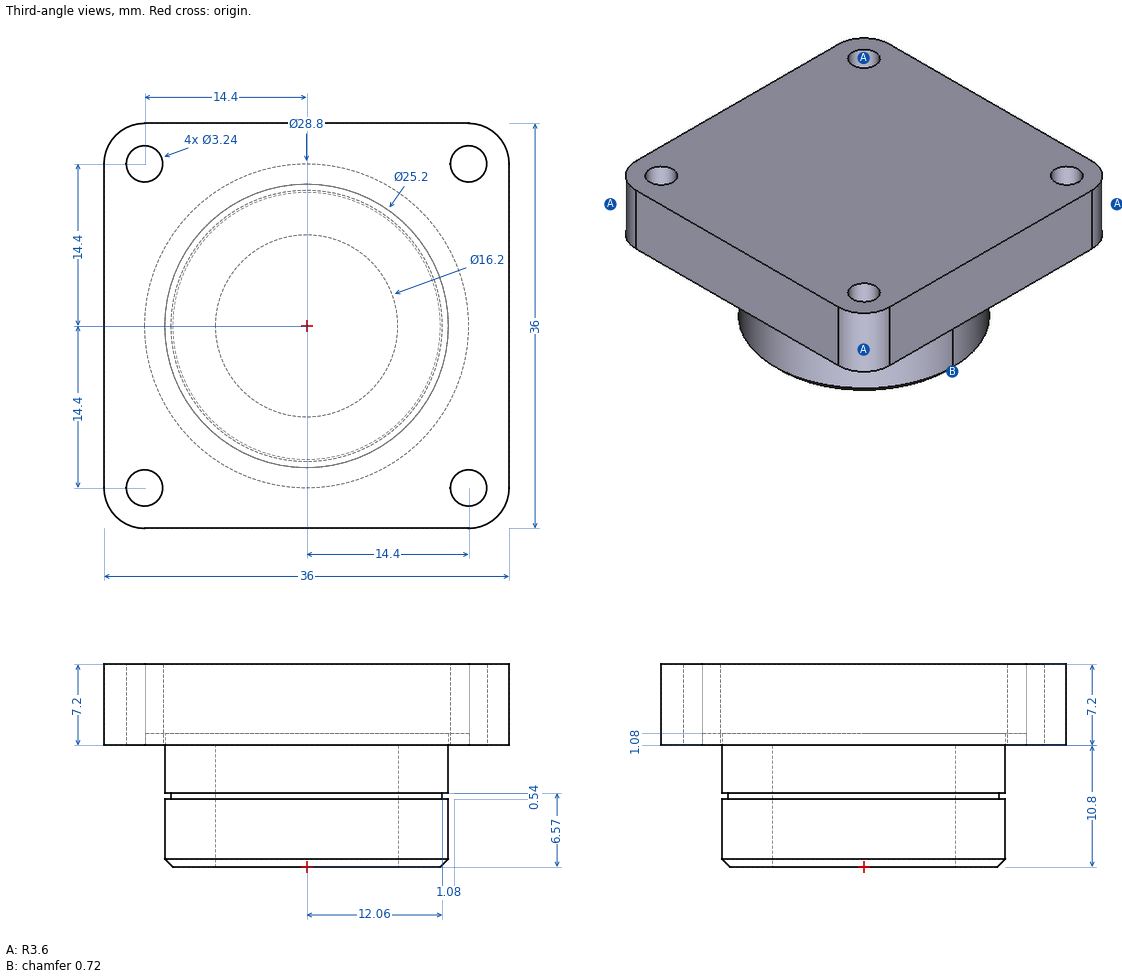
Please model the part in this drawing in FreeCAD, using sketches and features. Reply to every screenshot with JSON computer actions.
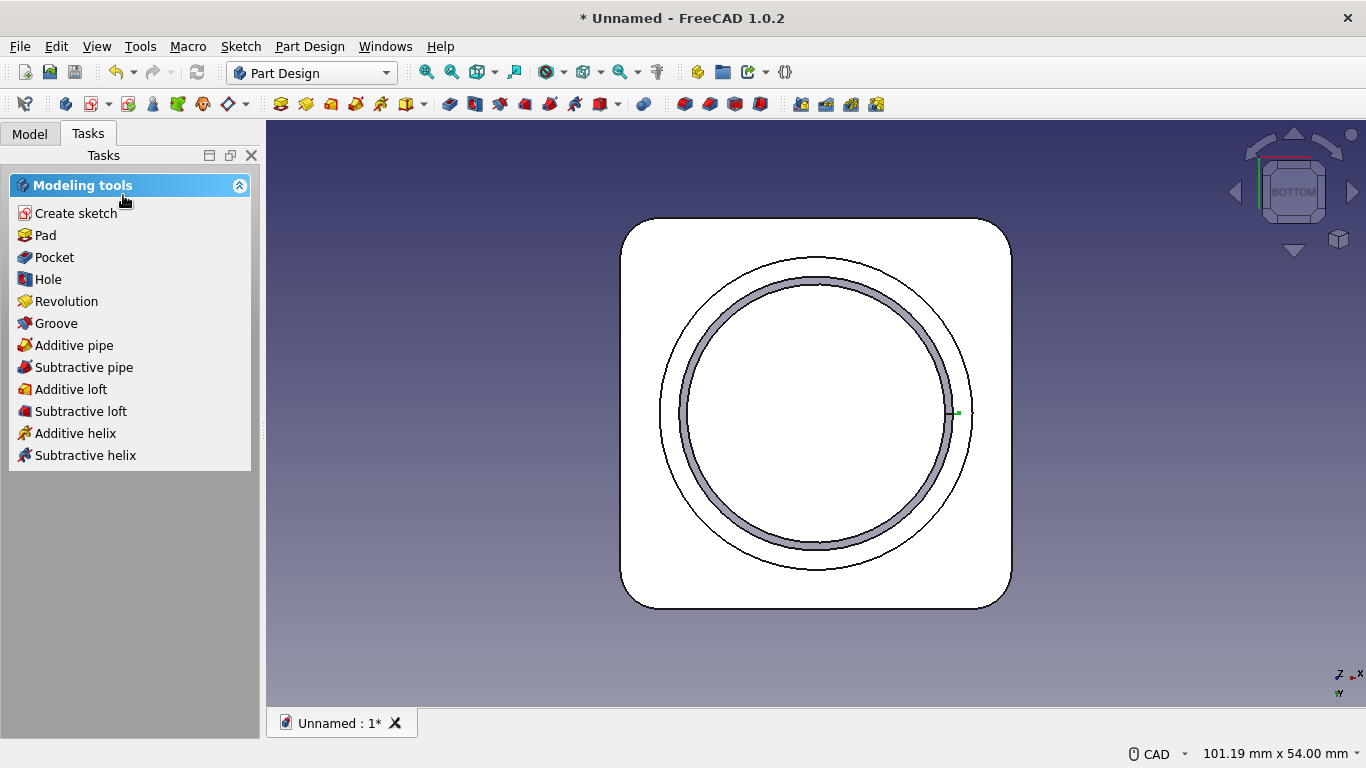
{"action": "left_click", "coordinate": [500, 104]}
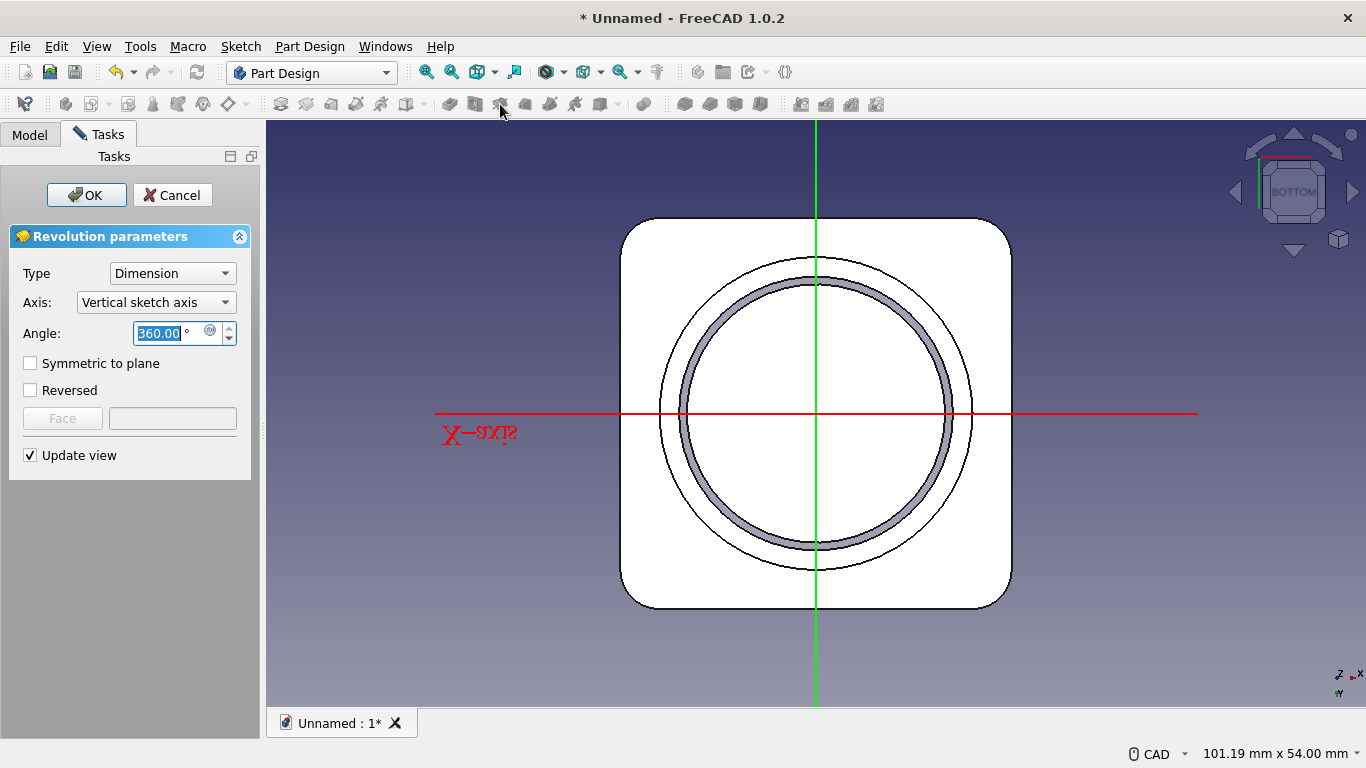
{"action": "left_click", "coordinate": [87, 195]}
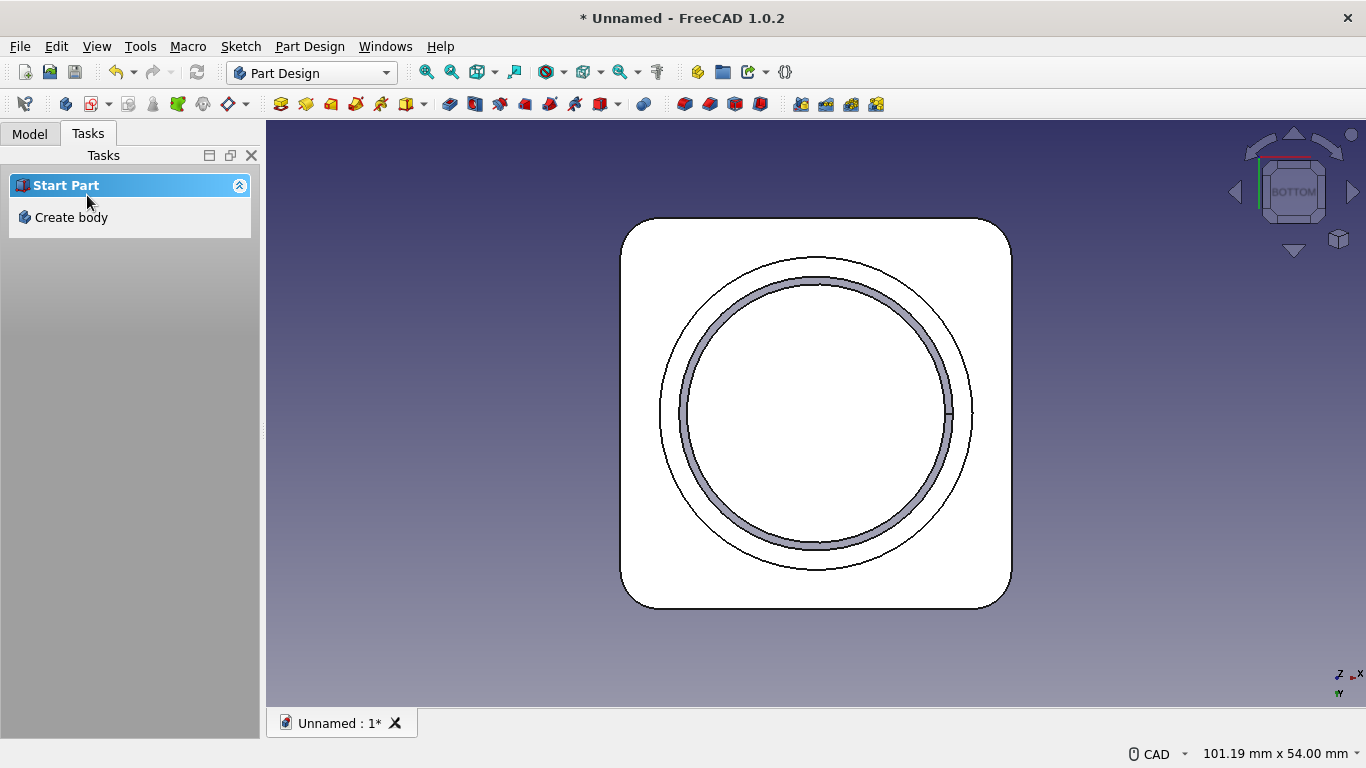
{"action": "left_click", "coordinate": [928, 245]}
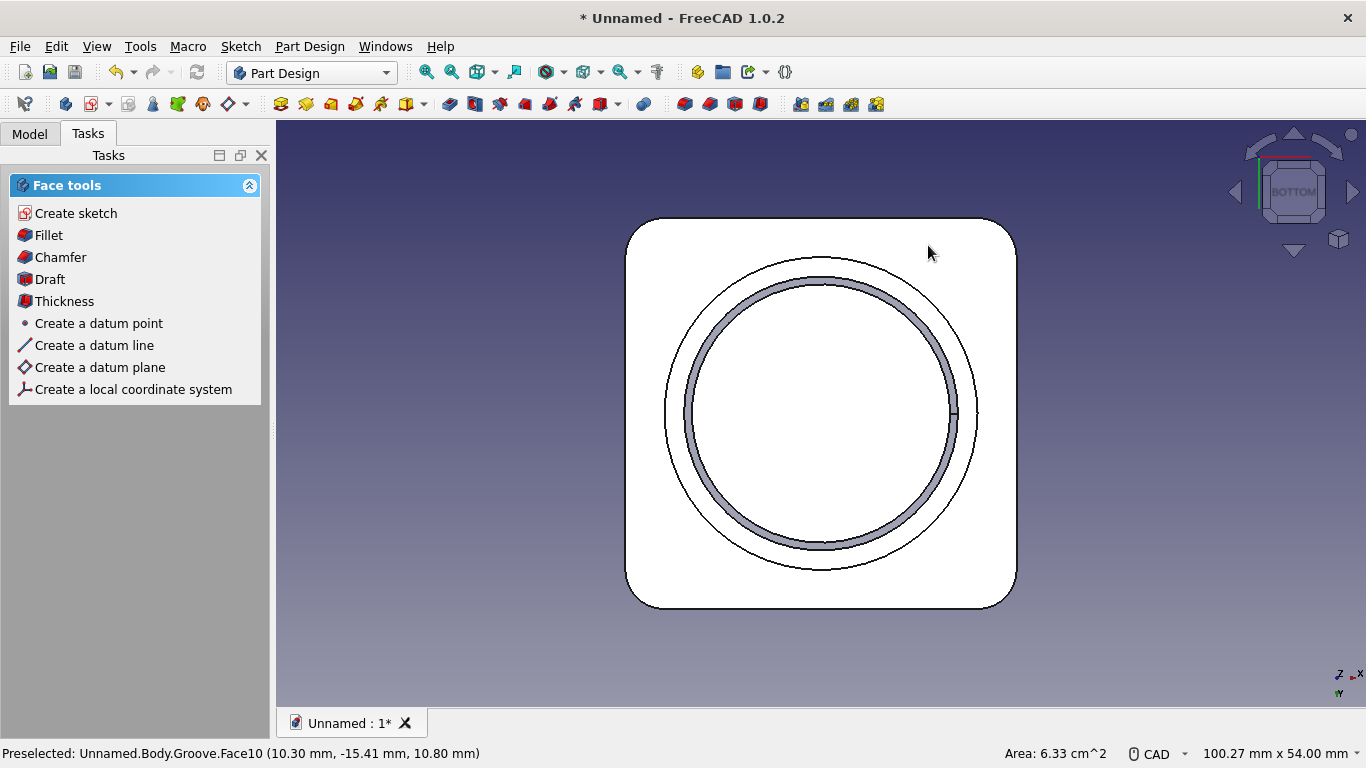
{"action": "left_click", "coordinate": [90, 104]}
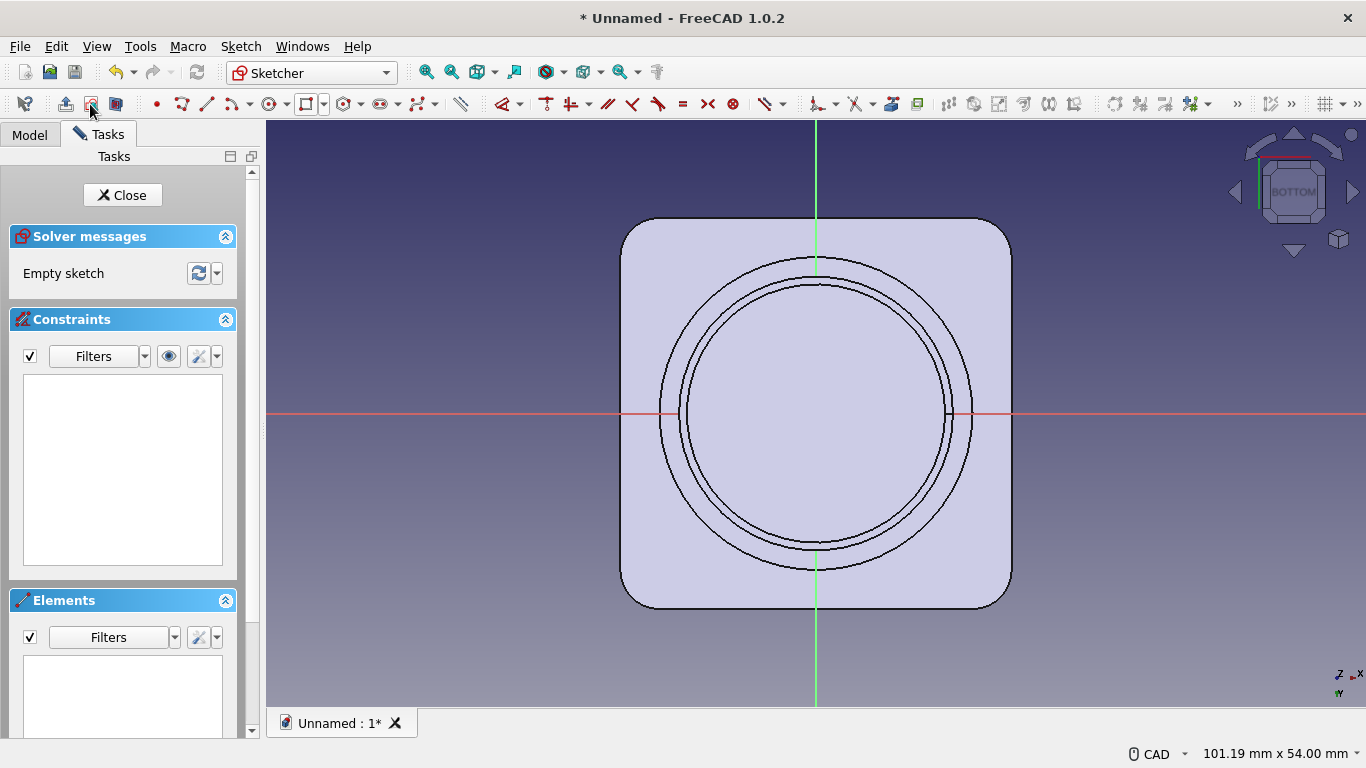
{"action": "left_click", "coordinate": [116, 104]}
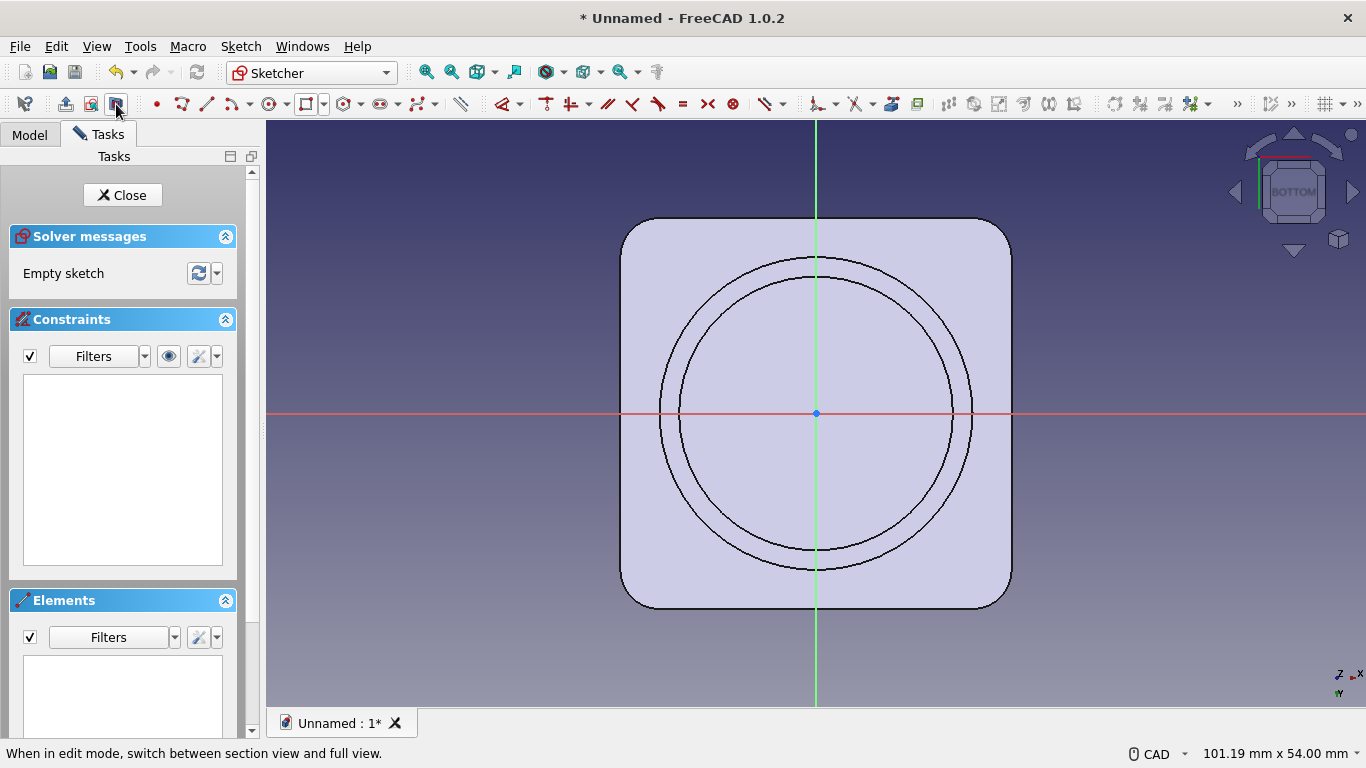
{"action": "left_click", "coordinate": [268, 104]}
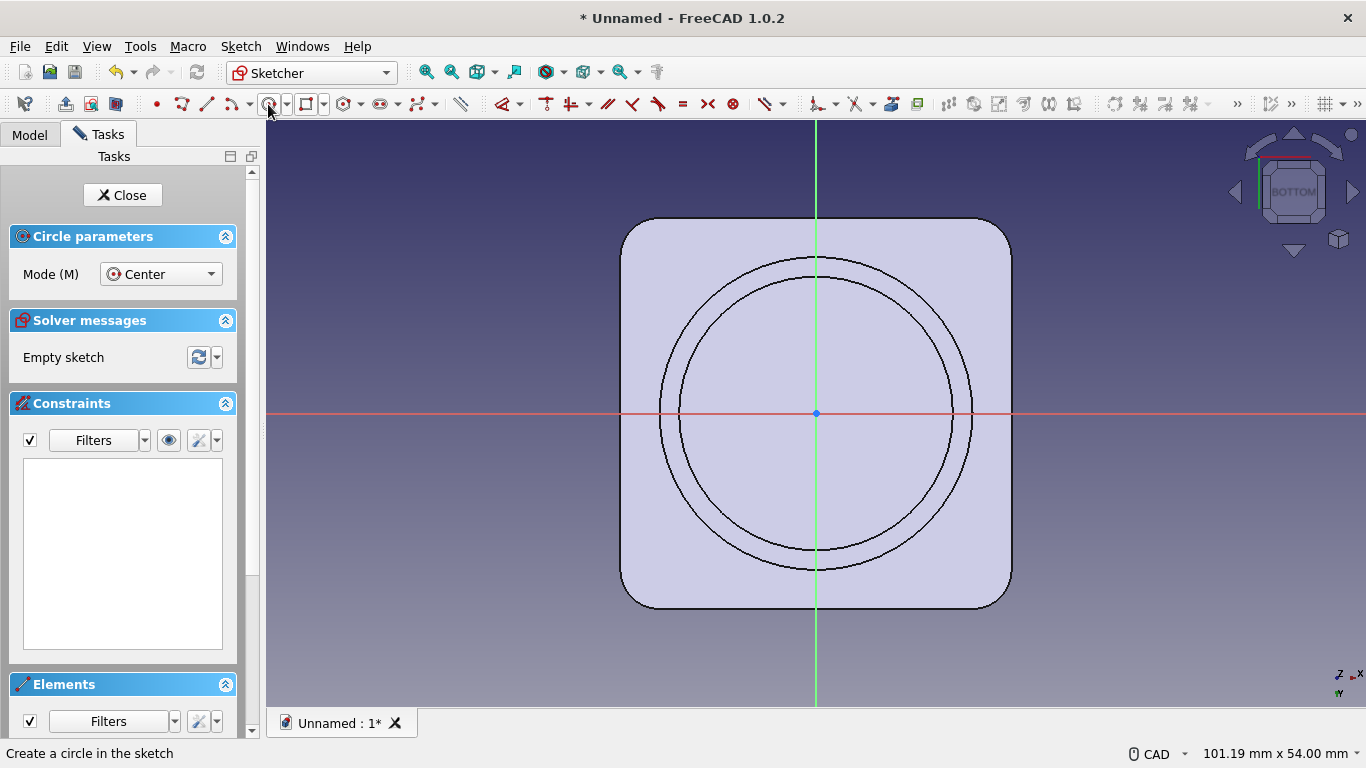
{"action": "scroll", "coordinate": [659, 570], "scroll_direction": "up", "scroll_amount": 2}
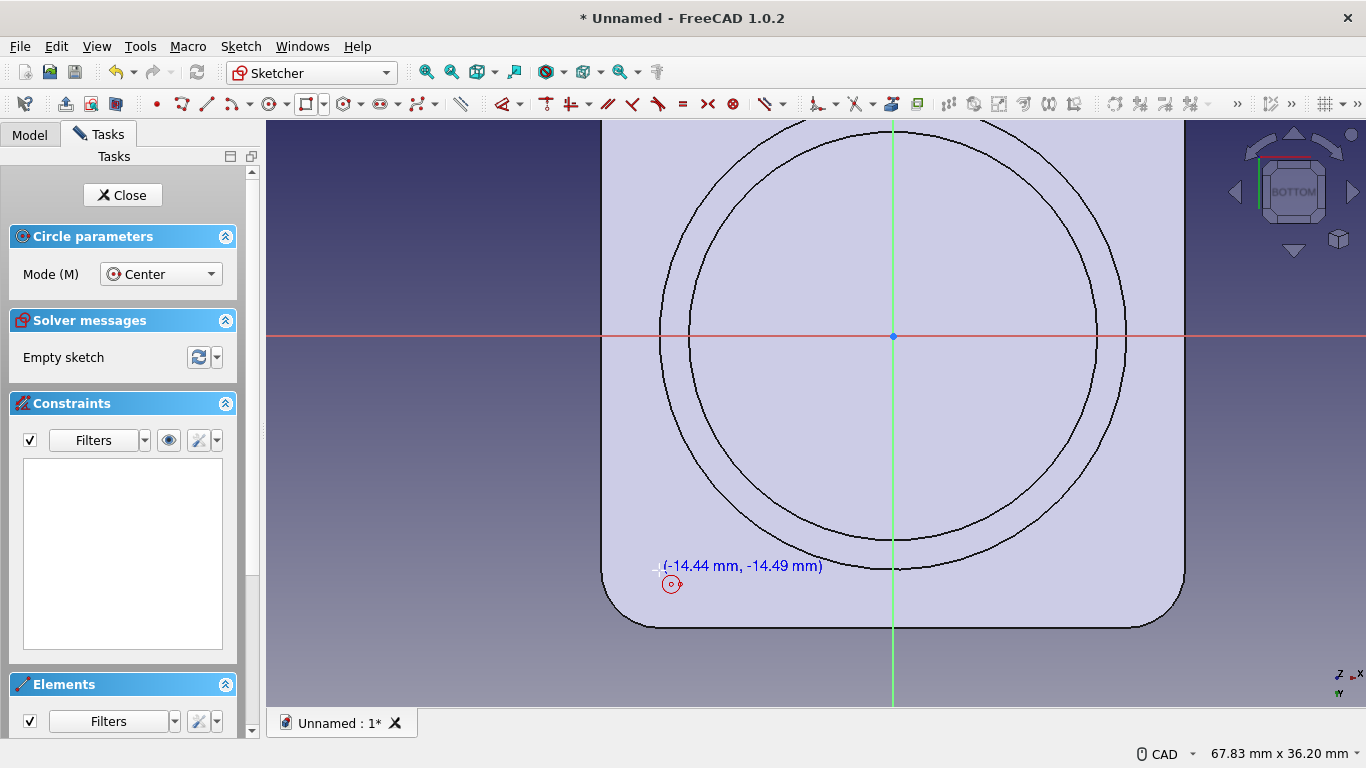
{"action": "left_click", "coordinate": [660, 570]}
{"action": "mouse_move", "coordinate": [678, 551]}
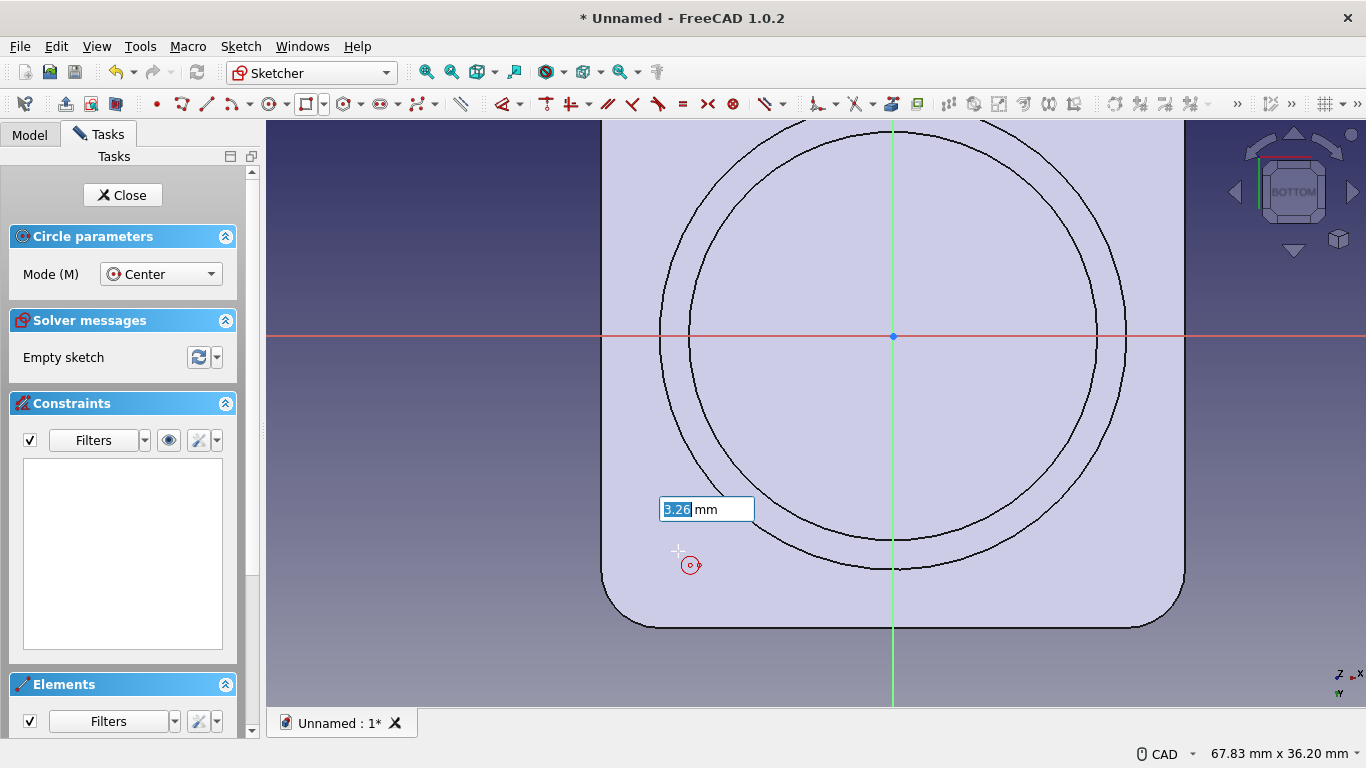
{"action": "type", "text": "3.24"}
{"action": "key", "text": "Return"}